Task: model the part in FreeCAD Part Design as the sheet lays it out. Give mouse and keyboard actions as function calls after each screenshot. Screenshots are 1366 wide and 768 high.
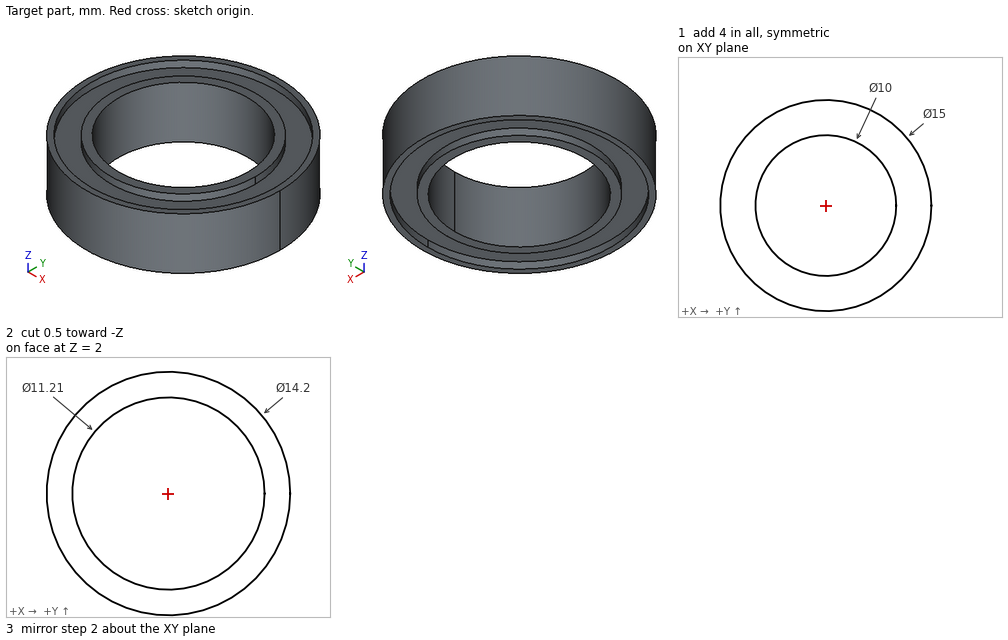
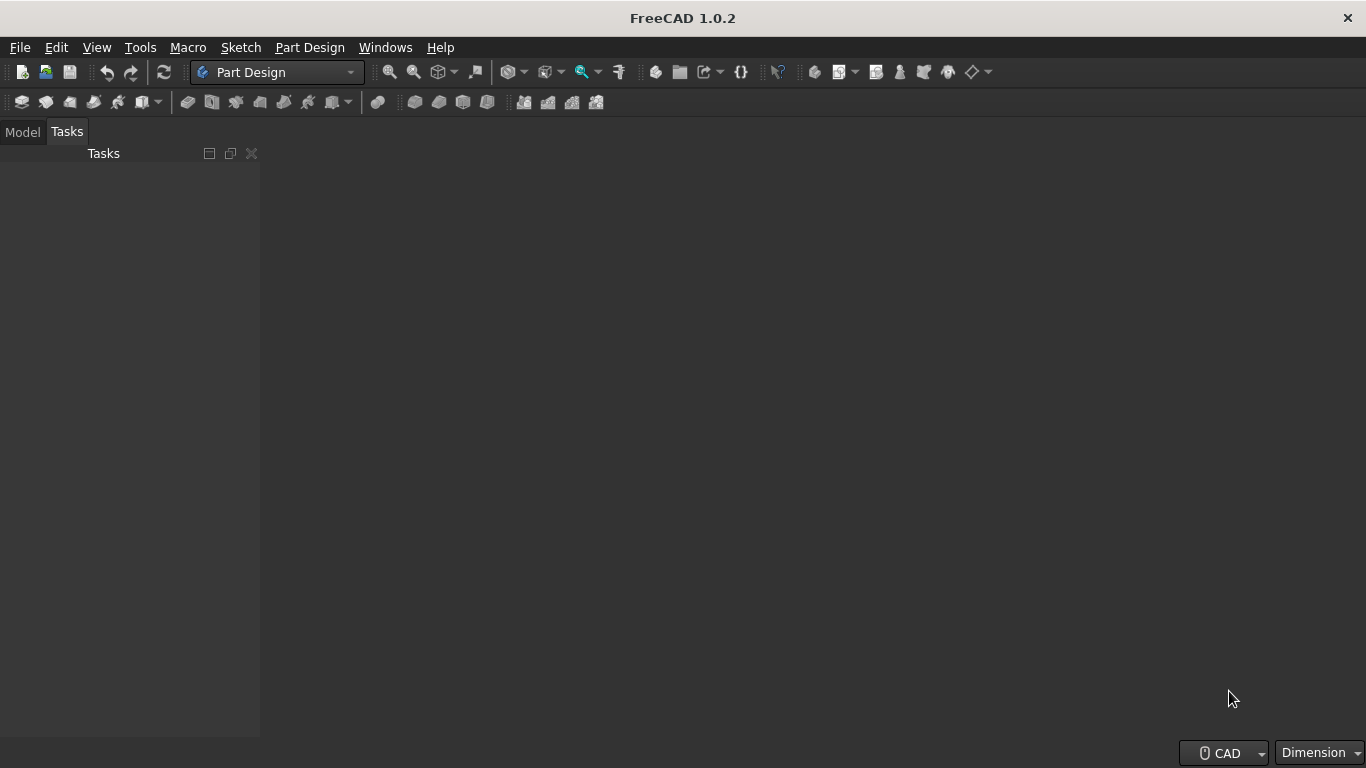
click(22, 72)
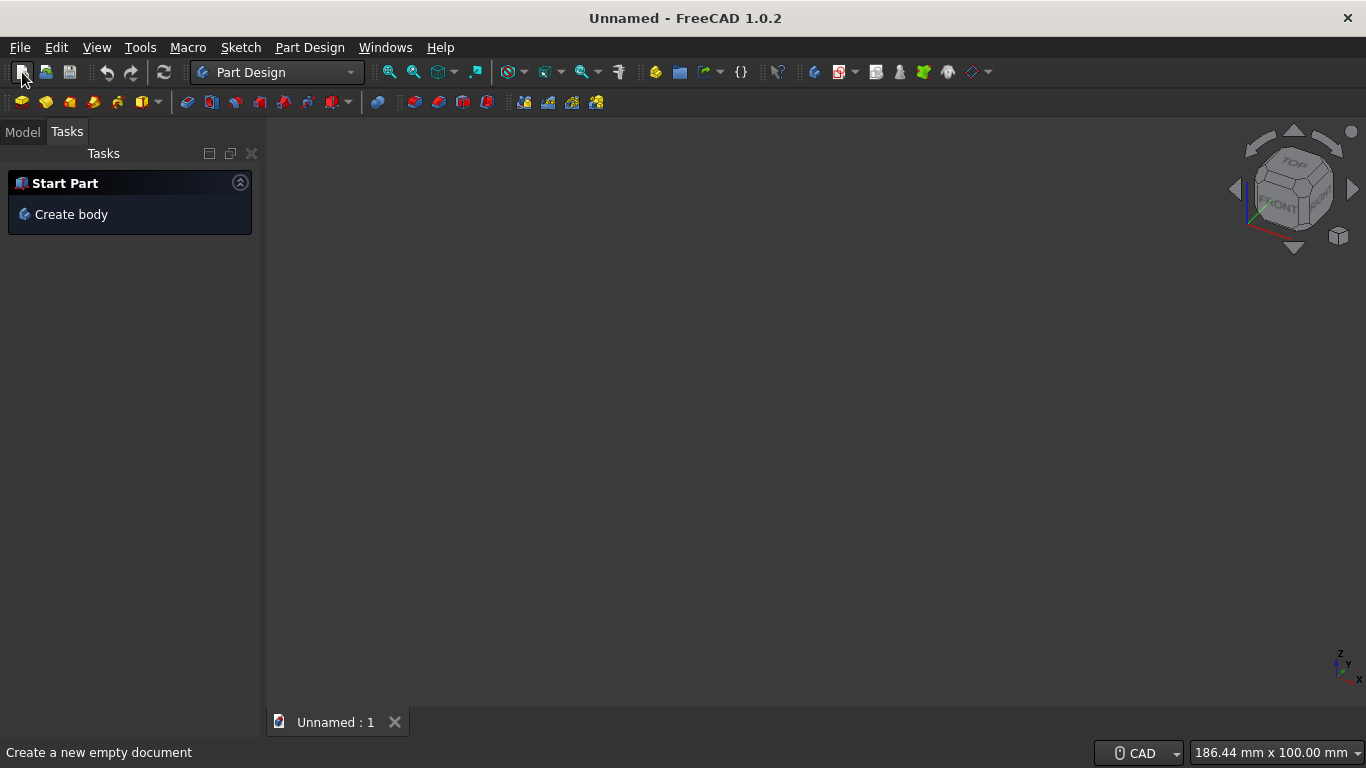
click(840, 72)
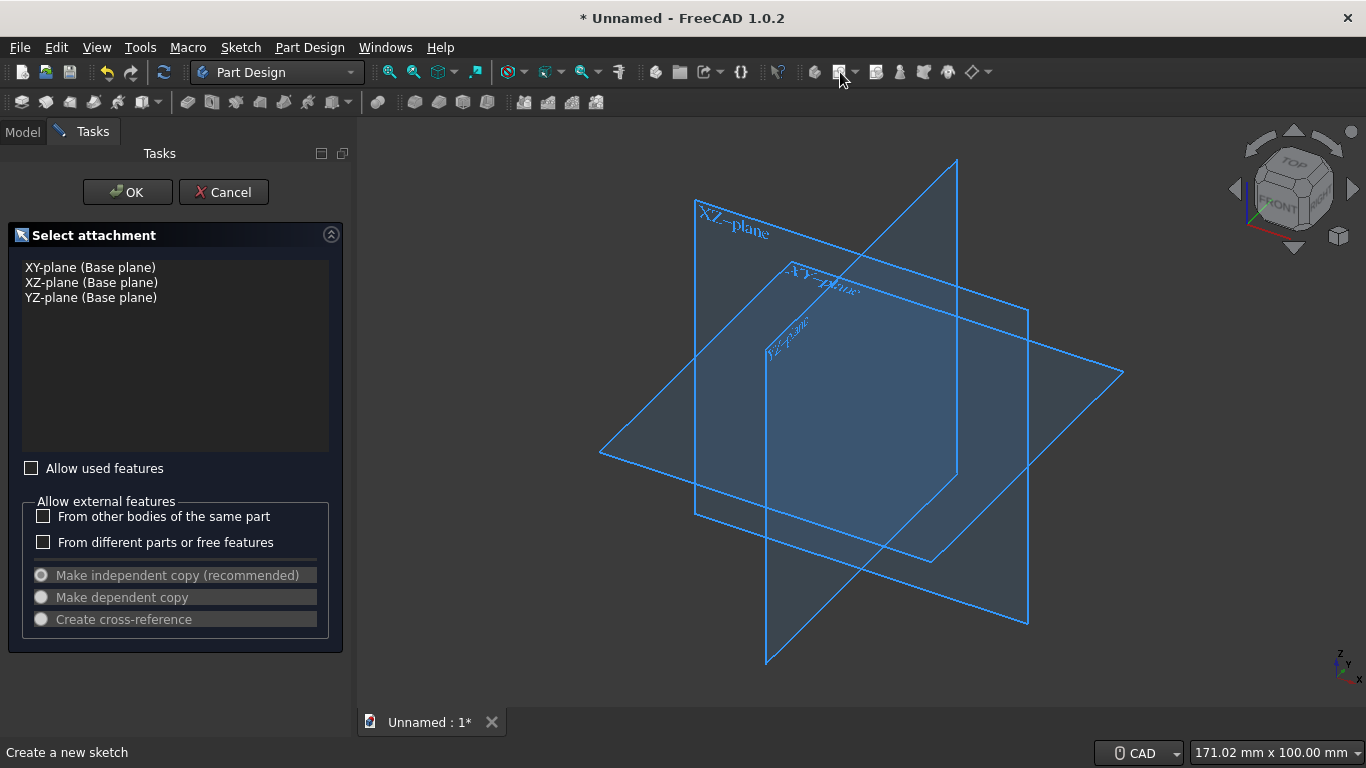
click(82, 268)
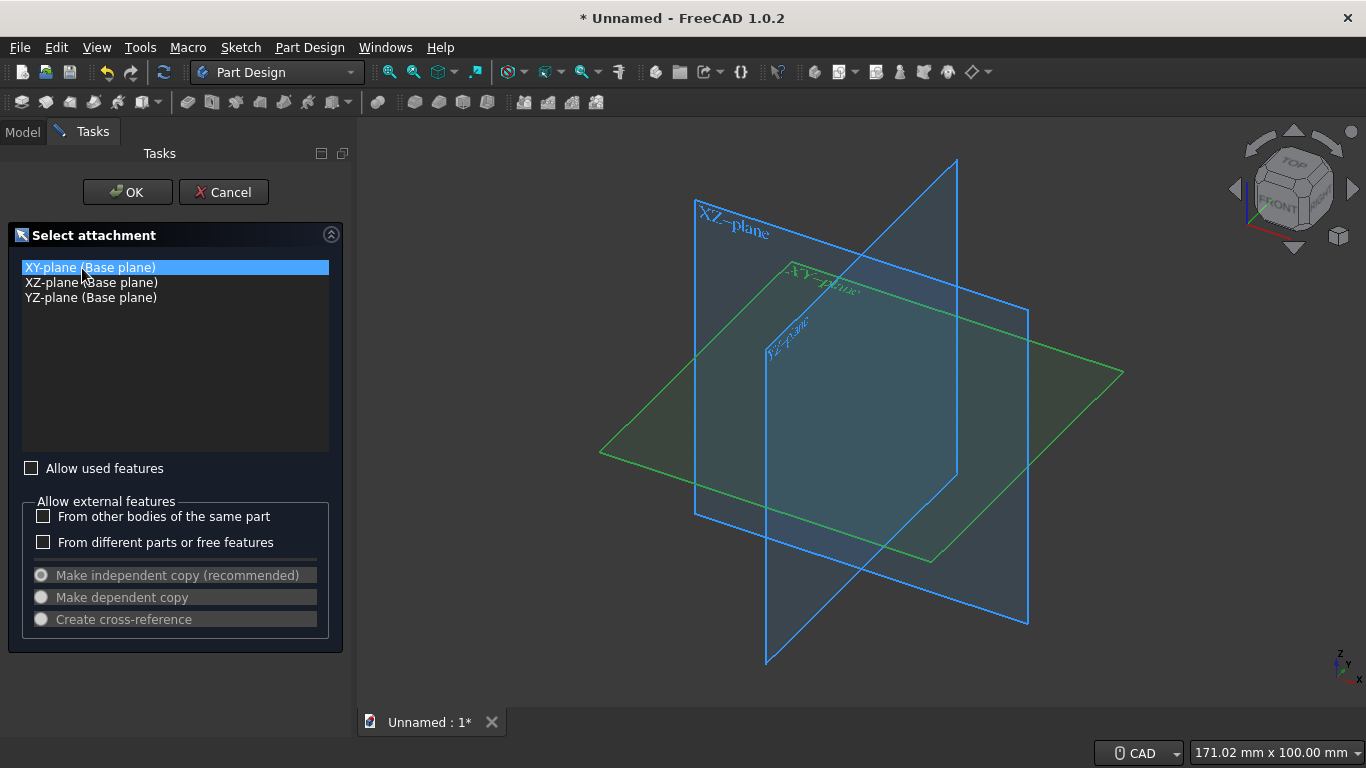
click(128, 192)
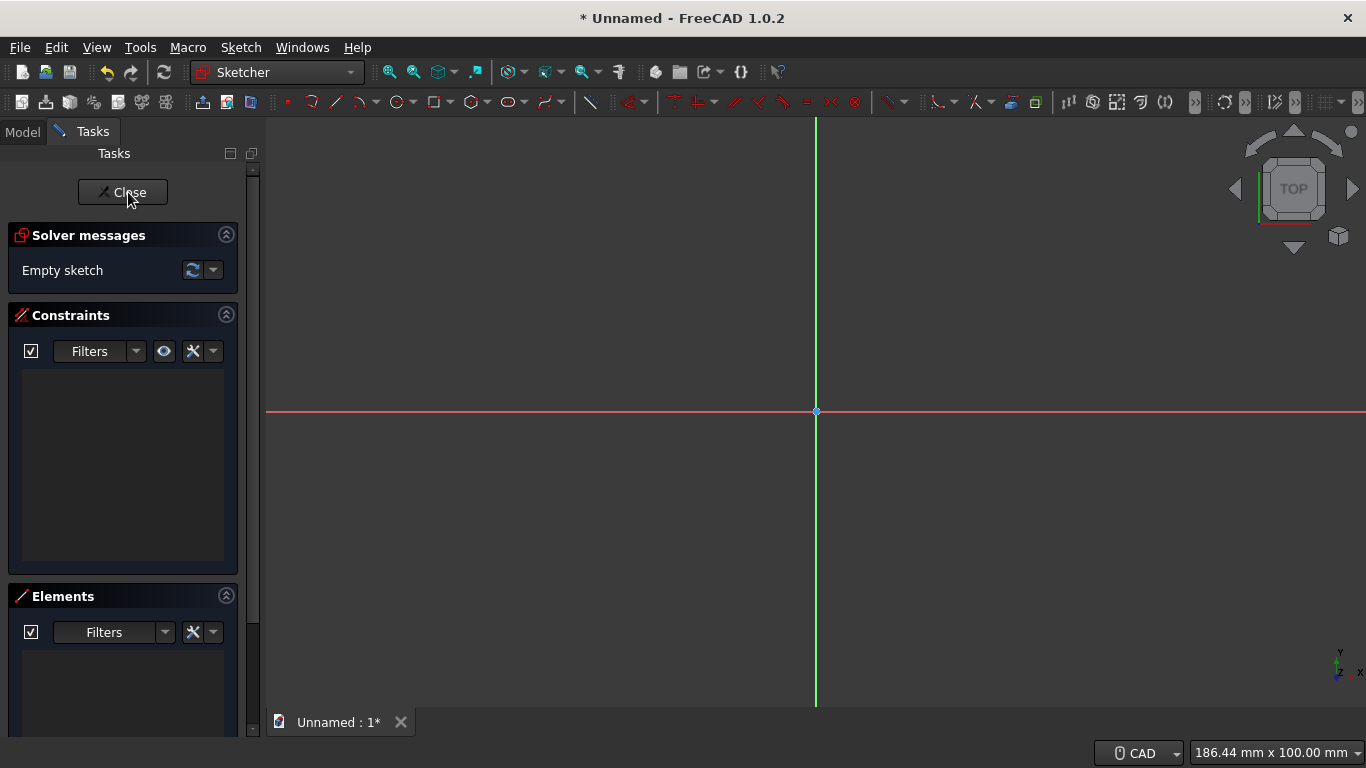
scroll(838, 412, up, 7)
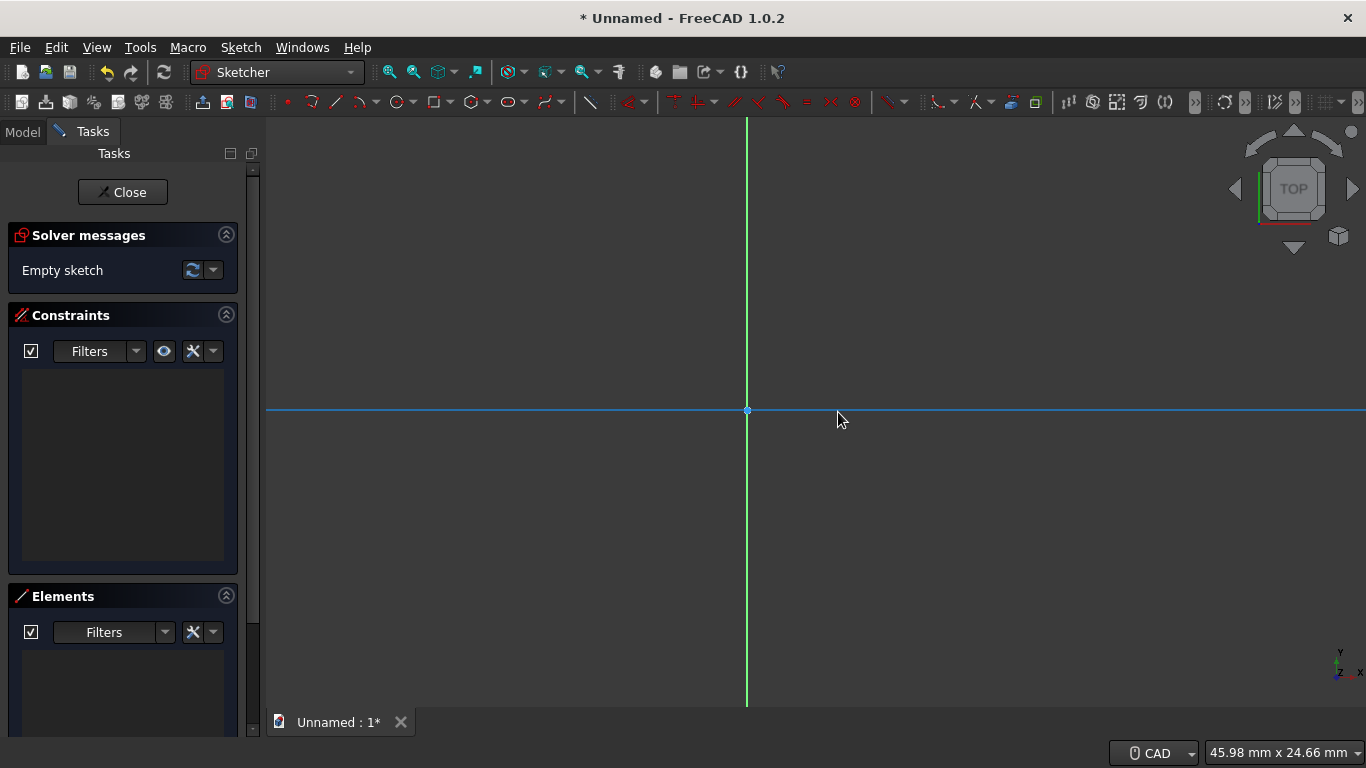
click(398, 102)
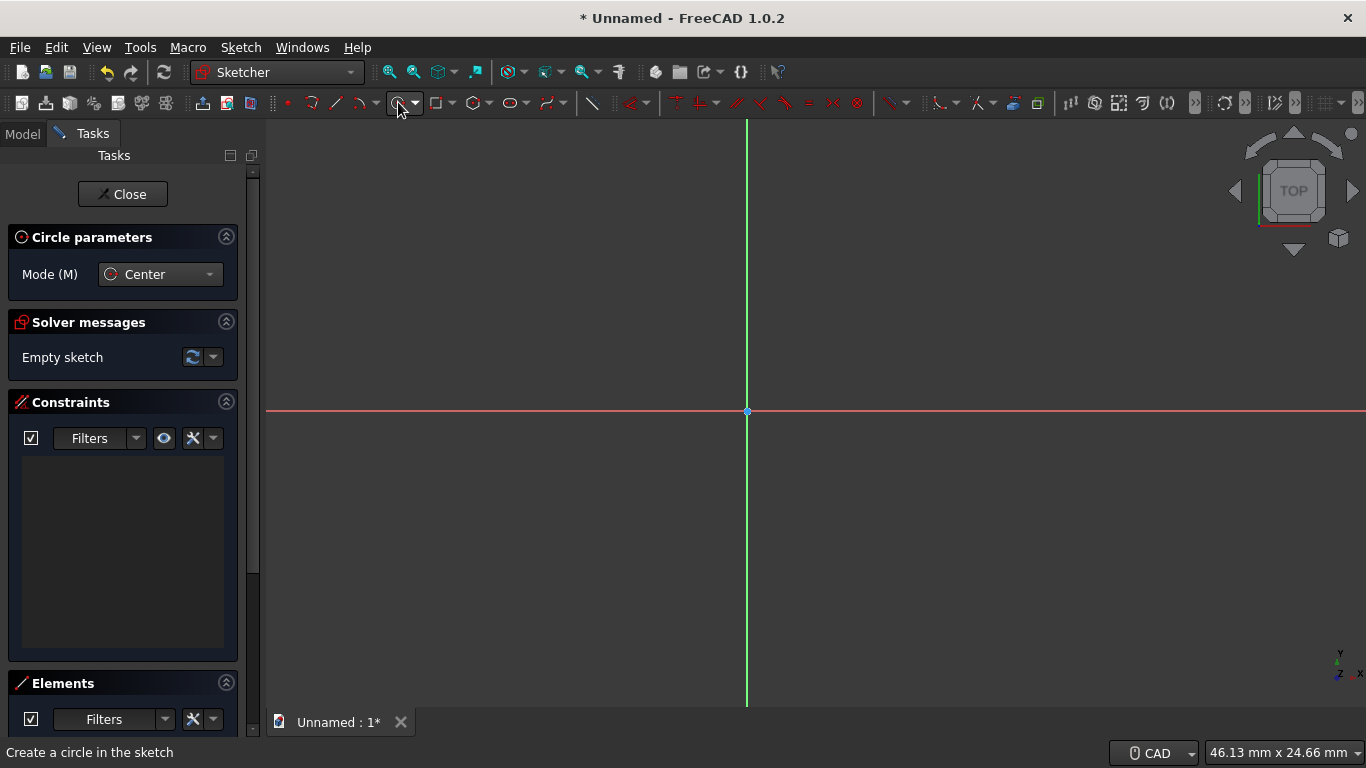
click(747, 411)
click(874, 285)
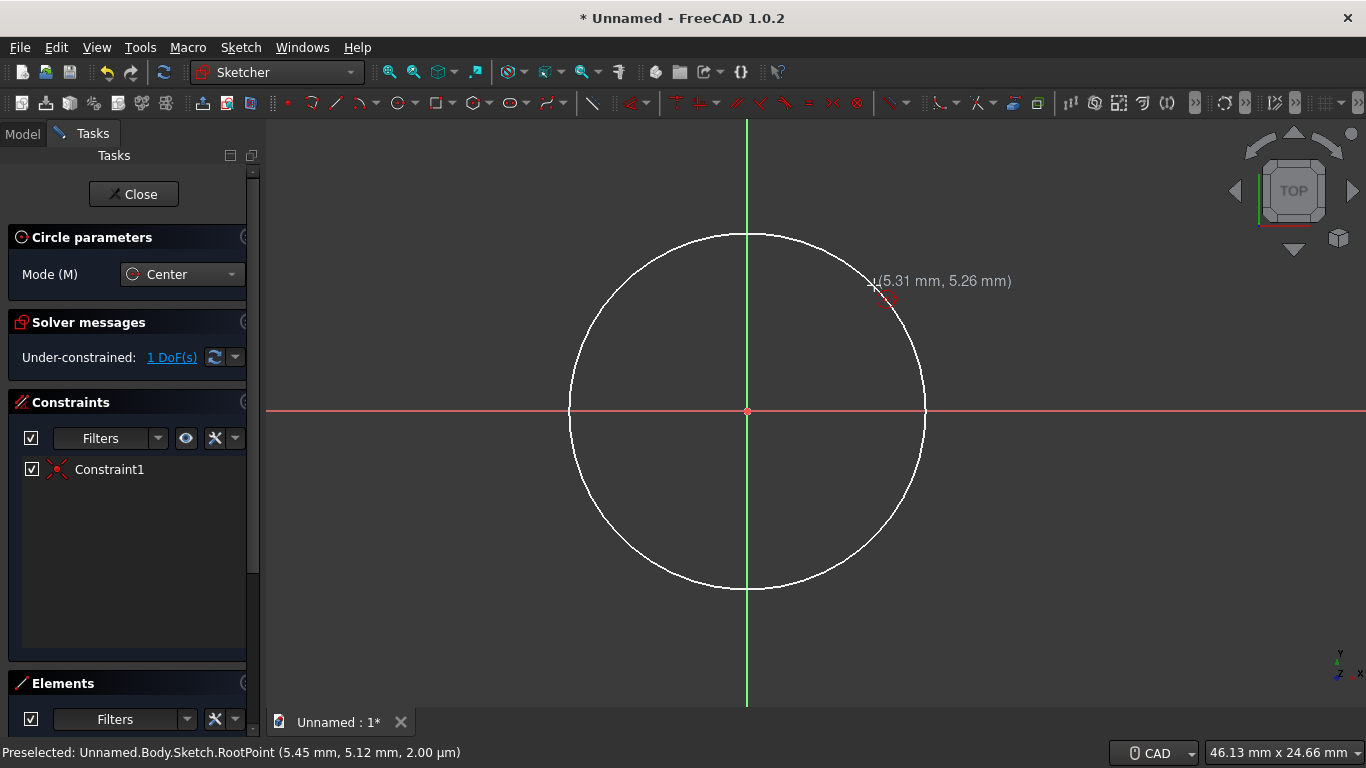
click(747, 411)
click(832, 327)
key(Escape)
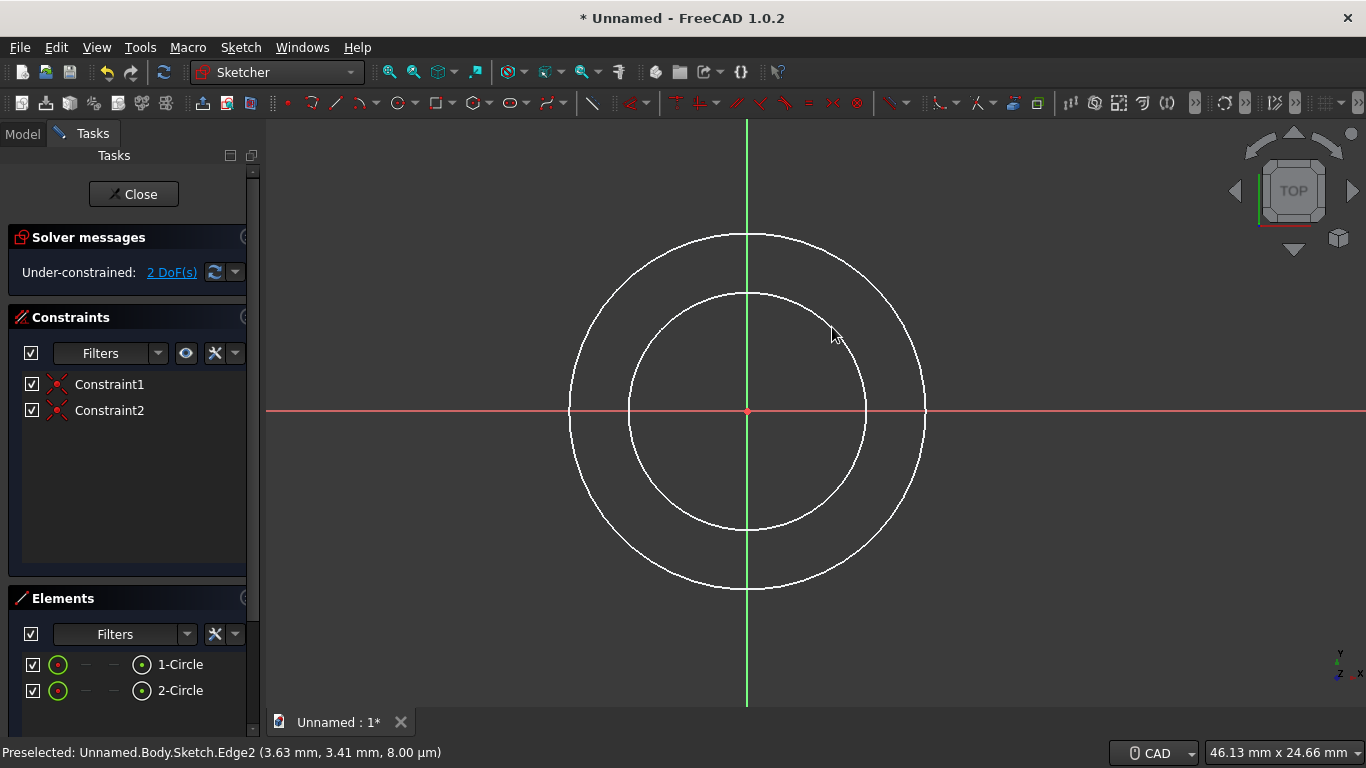
click(630, 104)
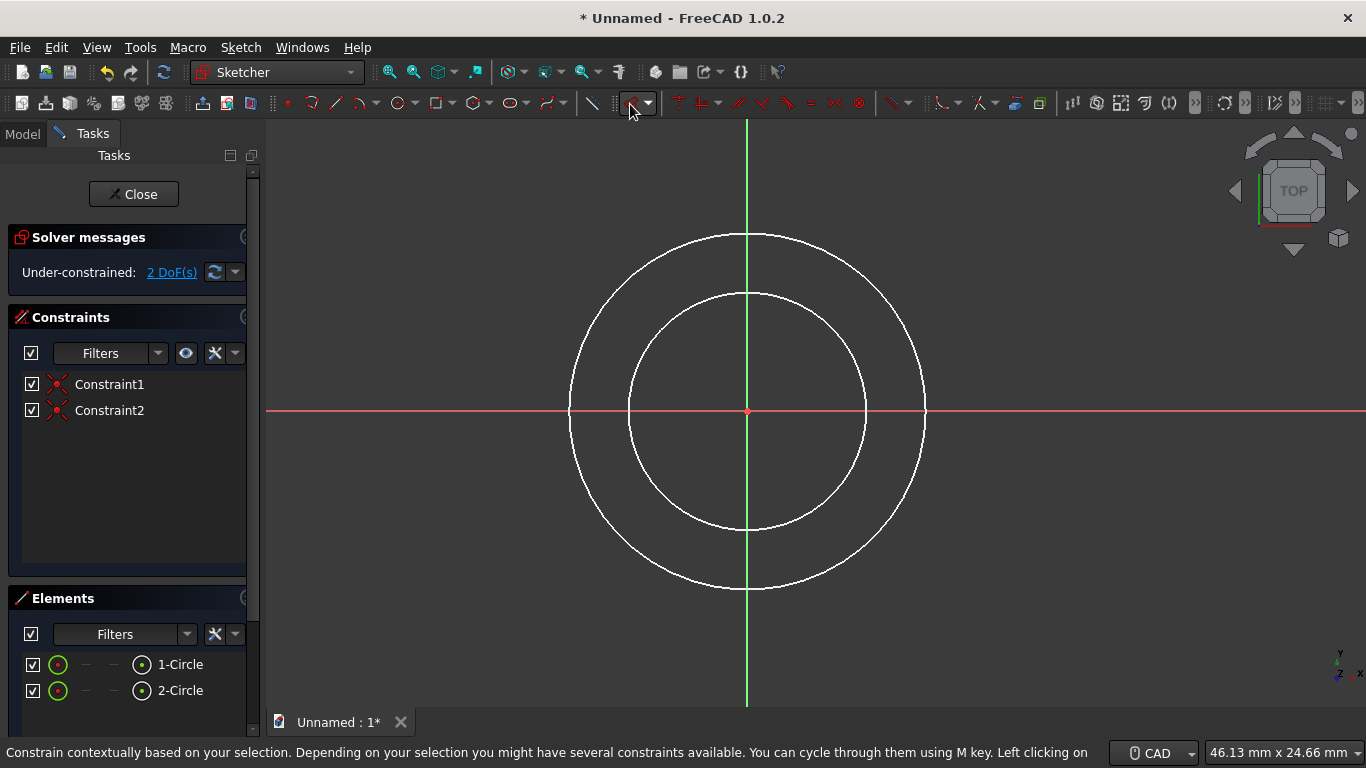
click(873, 285)
click(896, 262)